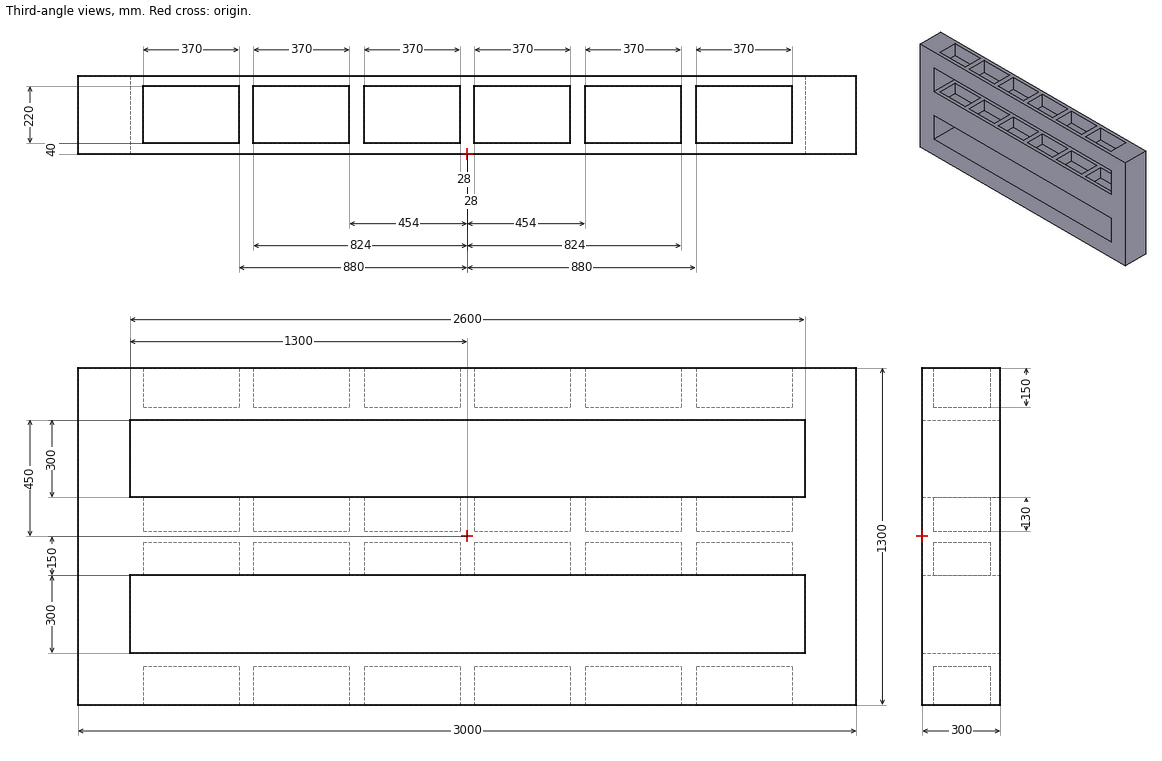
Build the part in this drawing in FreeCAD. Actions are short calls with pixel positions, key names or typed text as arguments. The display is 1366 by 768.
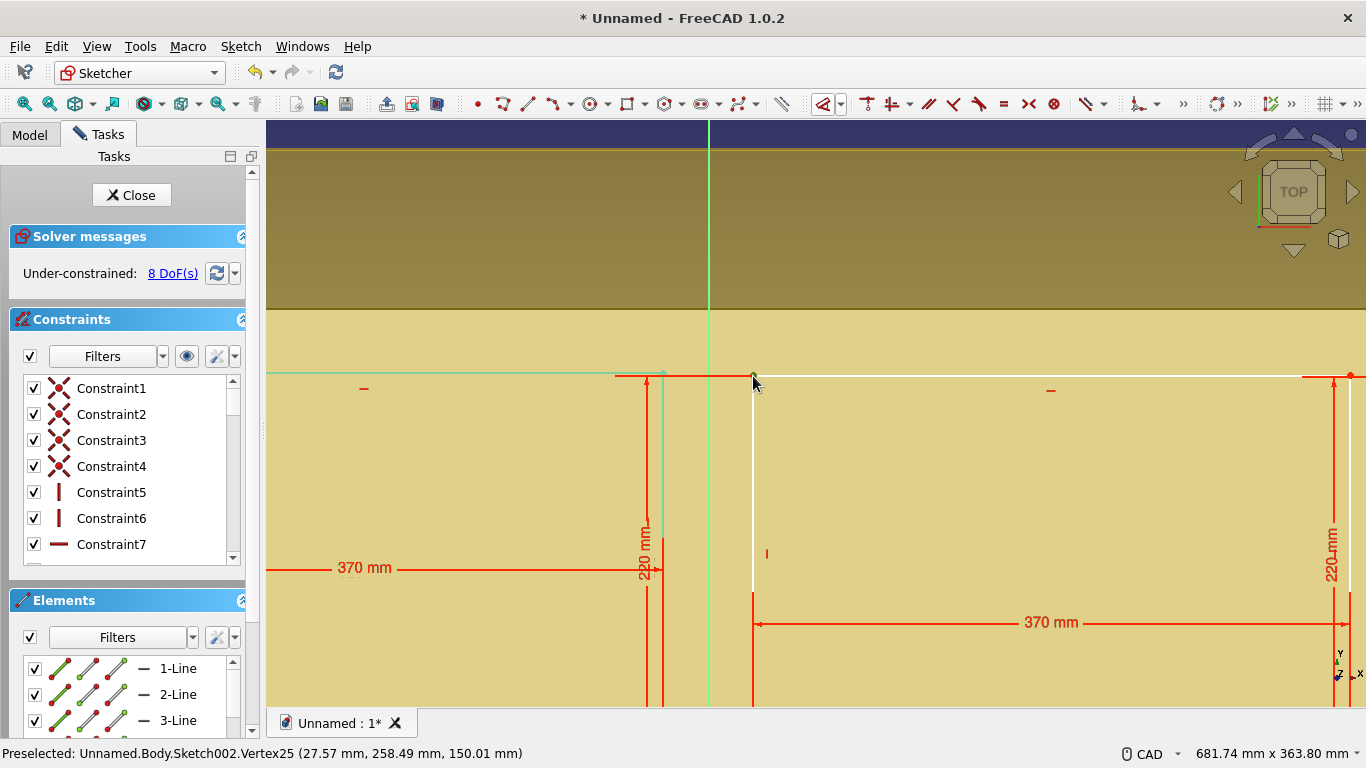
click(840, 104)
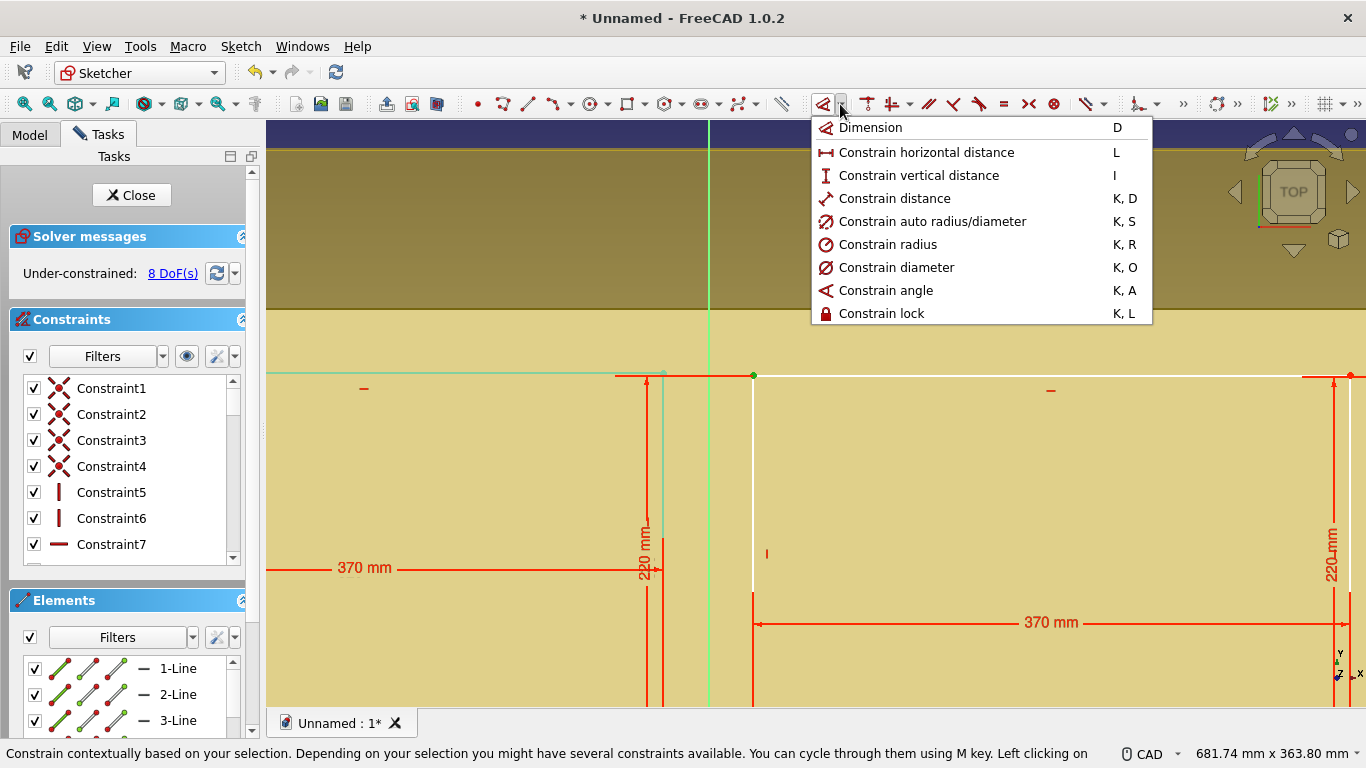
click(982, 152)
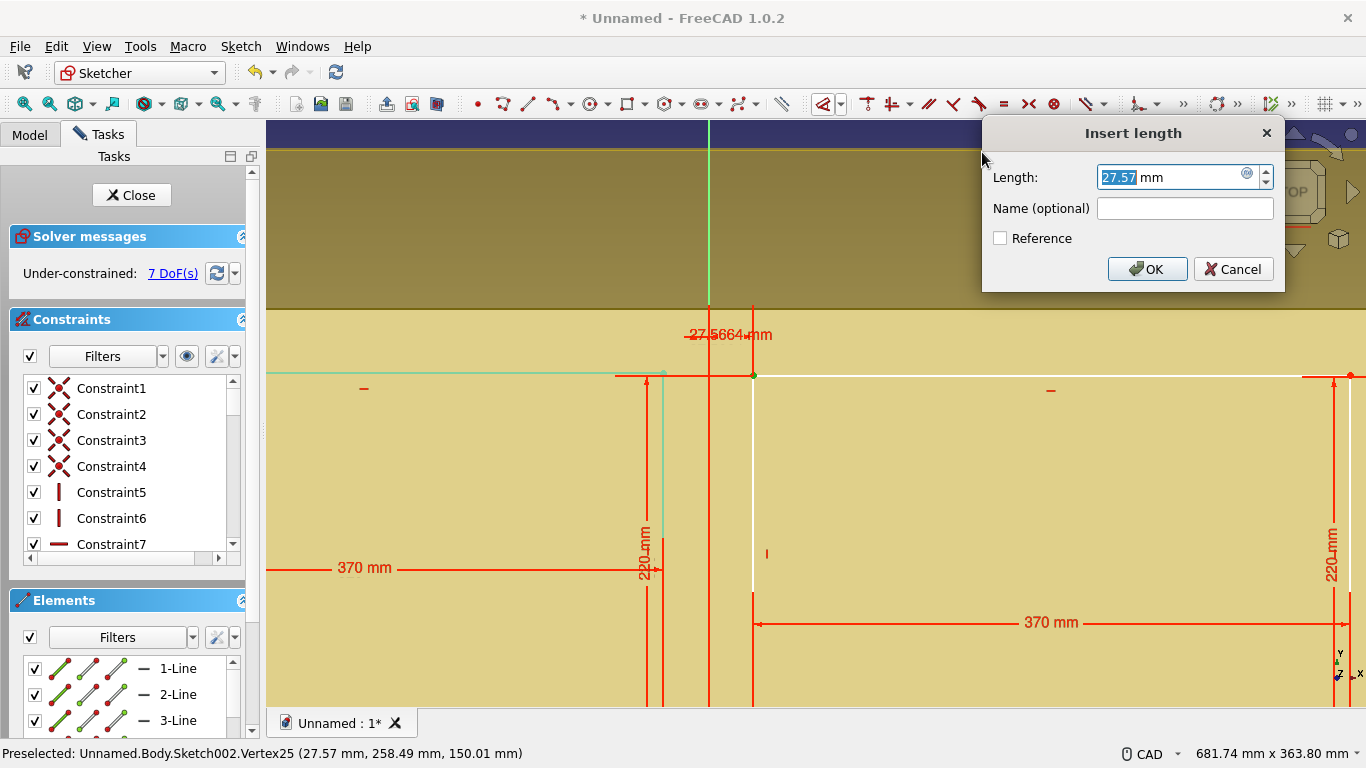
text(28)
key(Return)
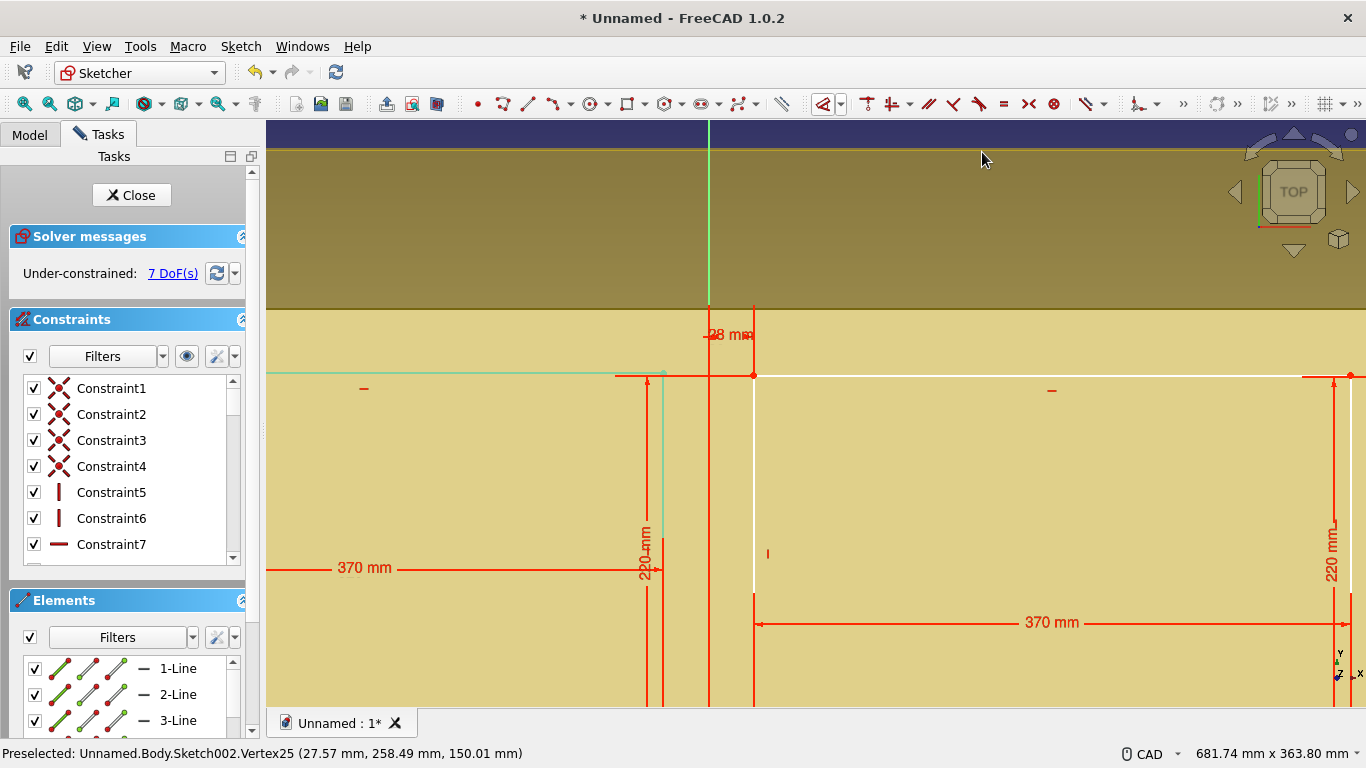
scroll(755, 380, down, 9)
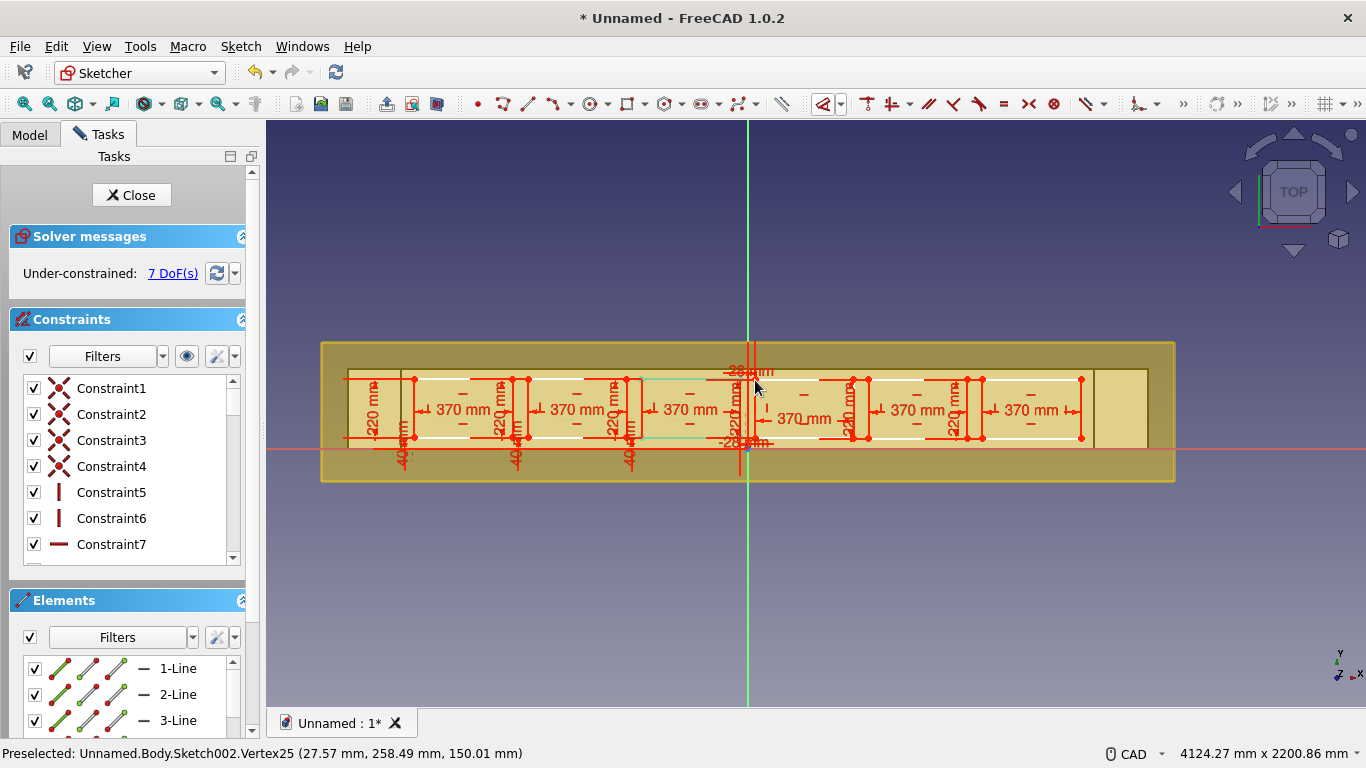
scroll(755, 438, up, 7)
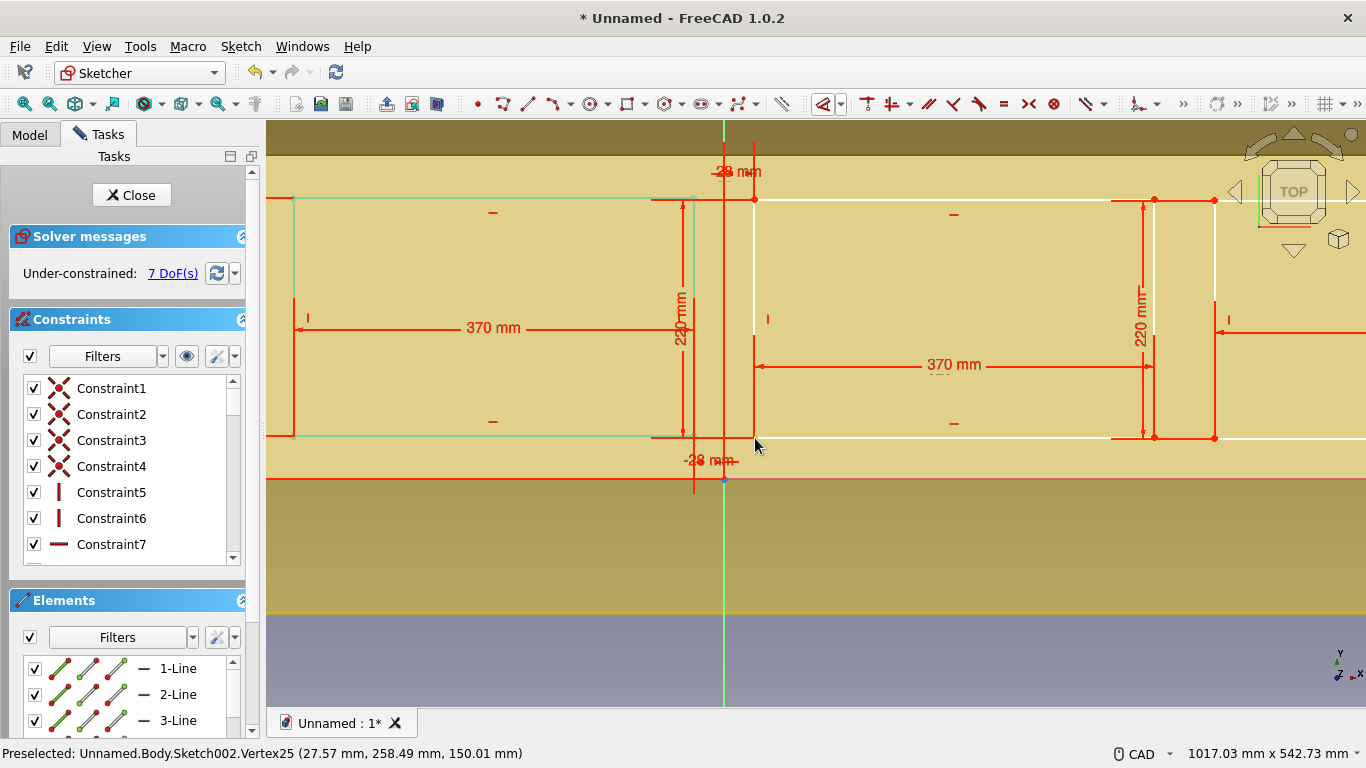
click(754, 438)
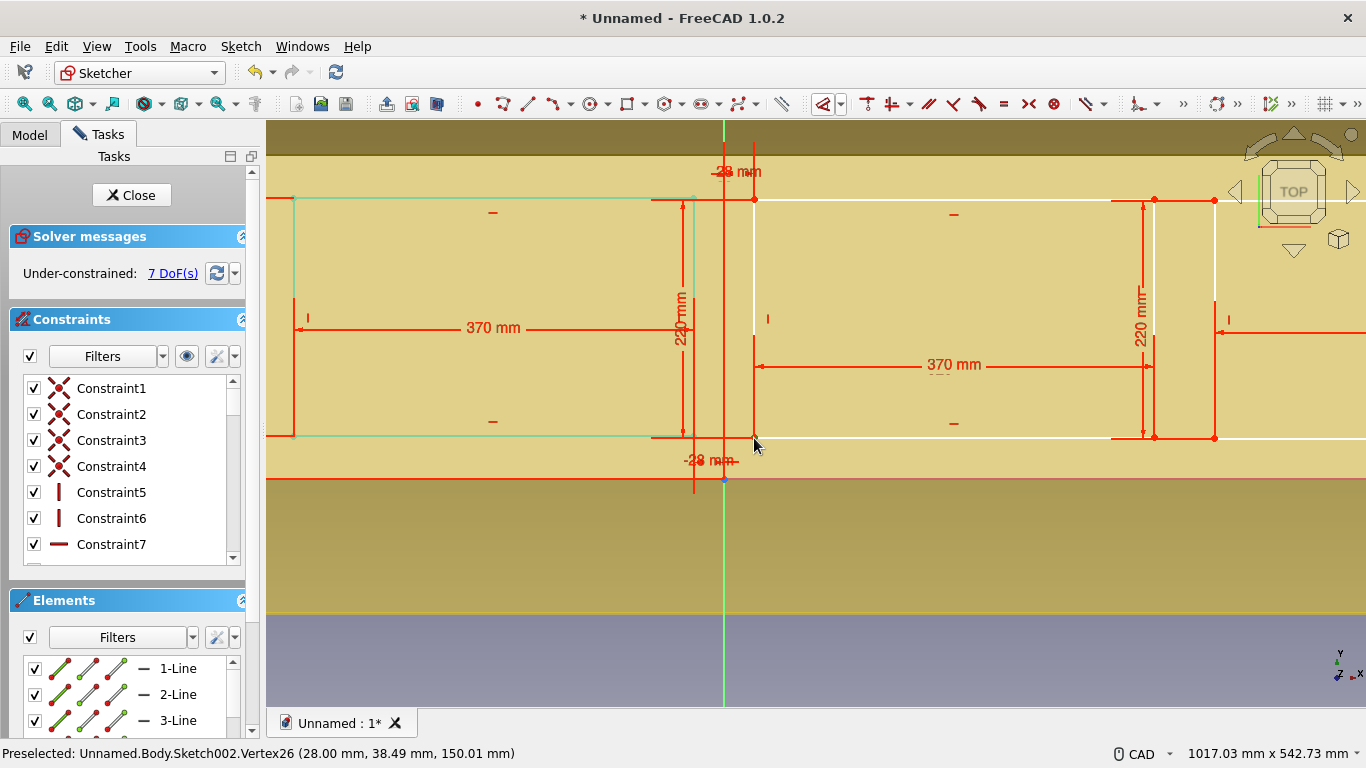
key(i)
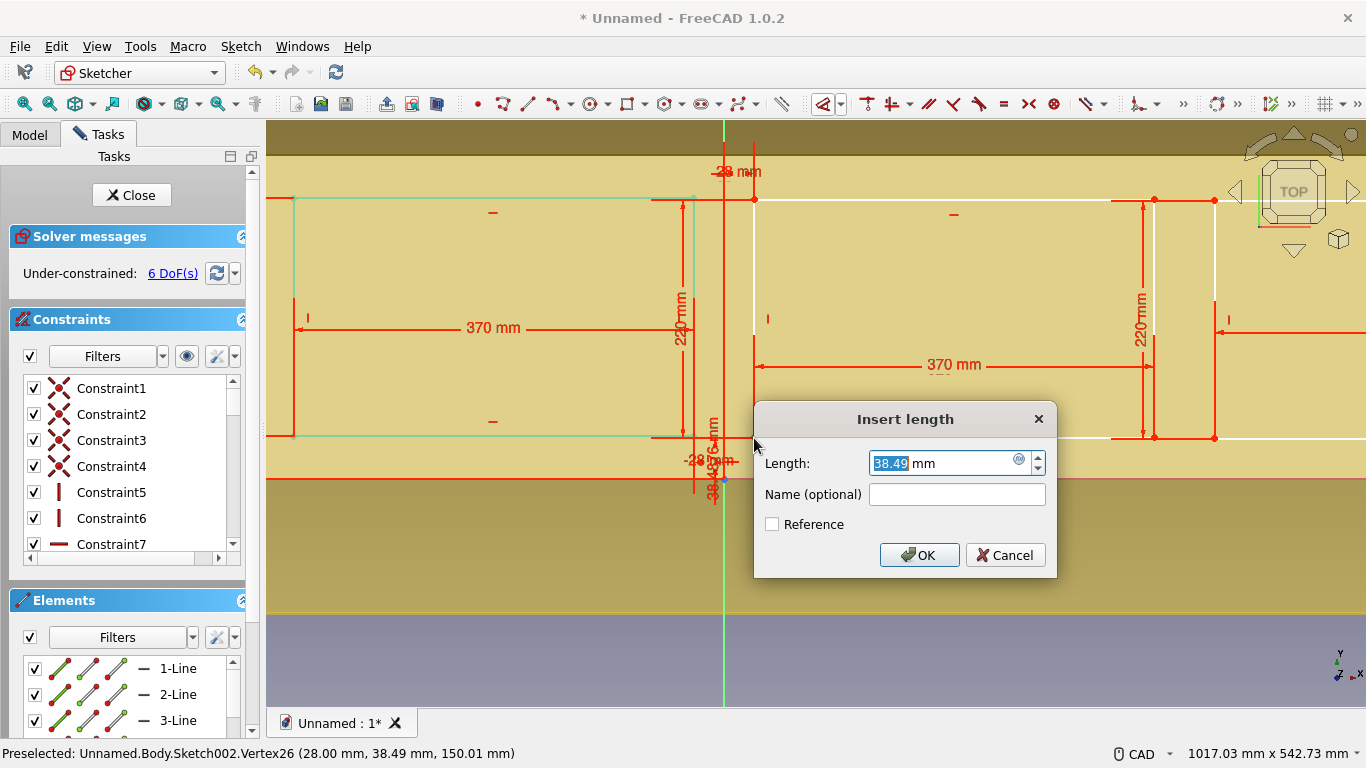
text(40)
key(Return)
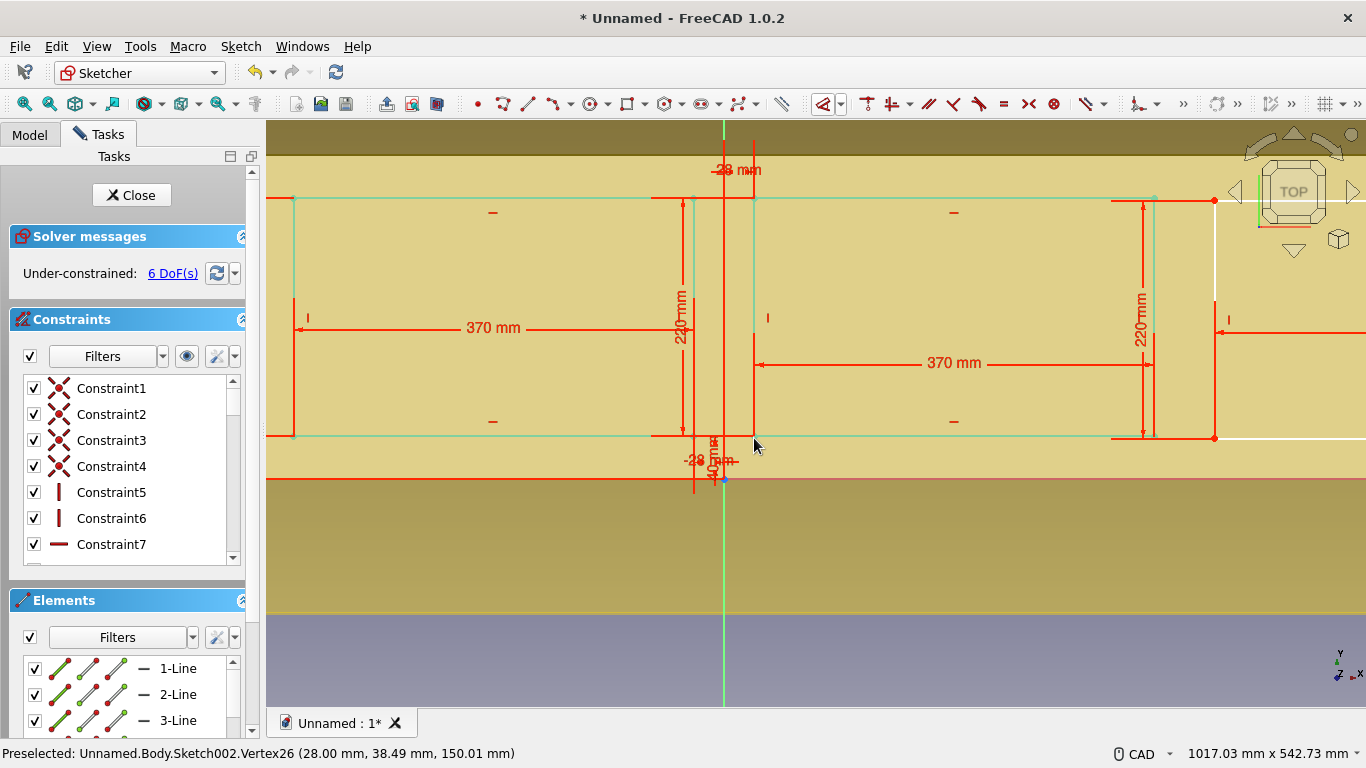
scroll(755, 438, down, 7)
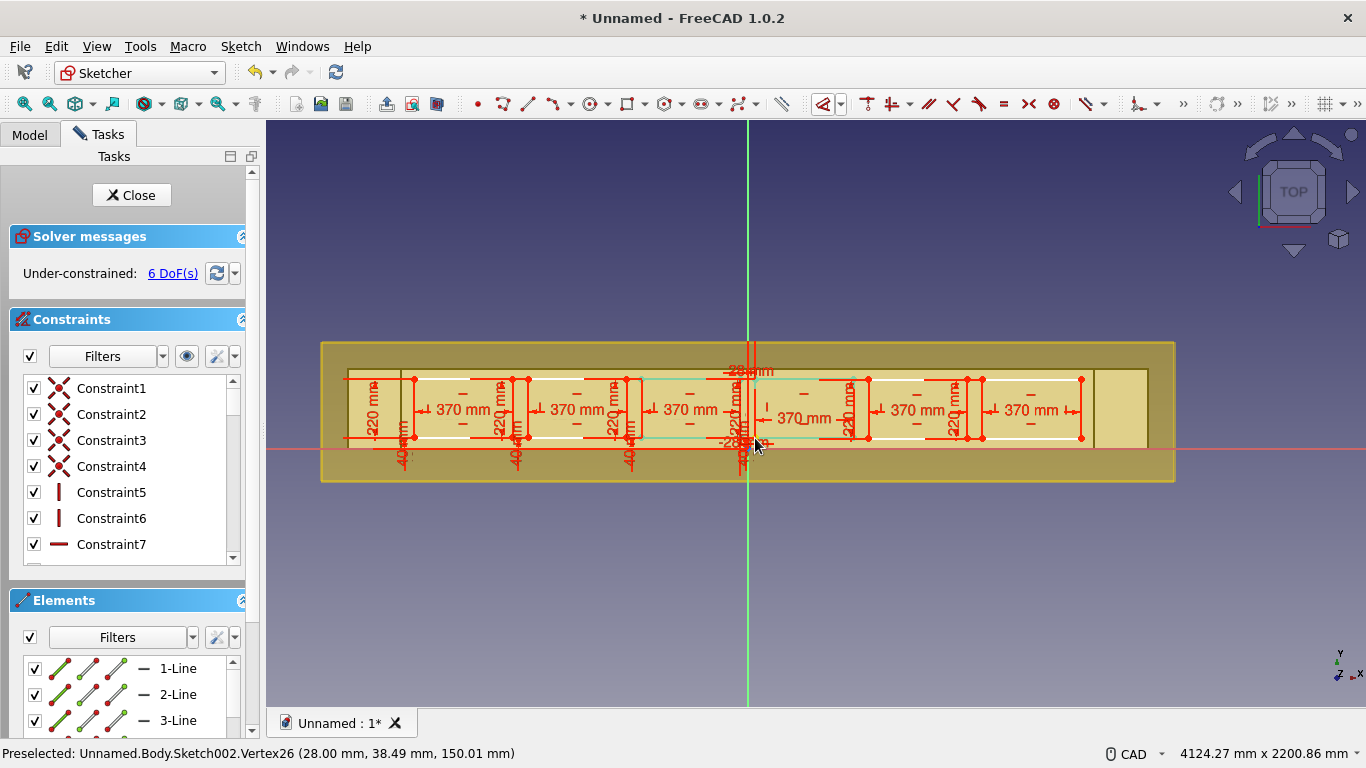
scroll(869, 439, up, 7)